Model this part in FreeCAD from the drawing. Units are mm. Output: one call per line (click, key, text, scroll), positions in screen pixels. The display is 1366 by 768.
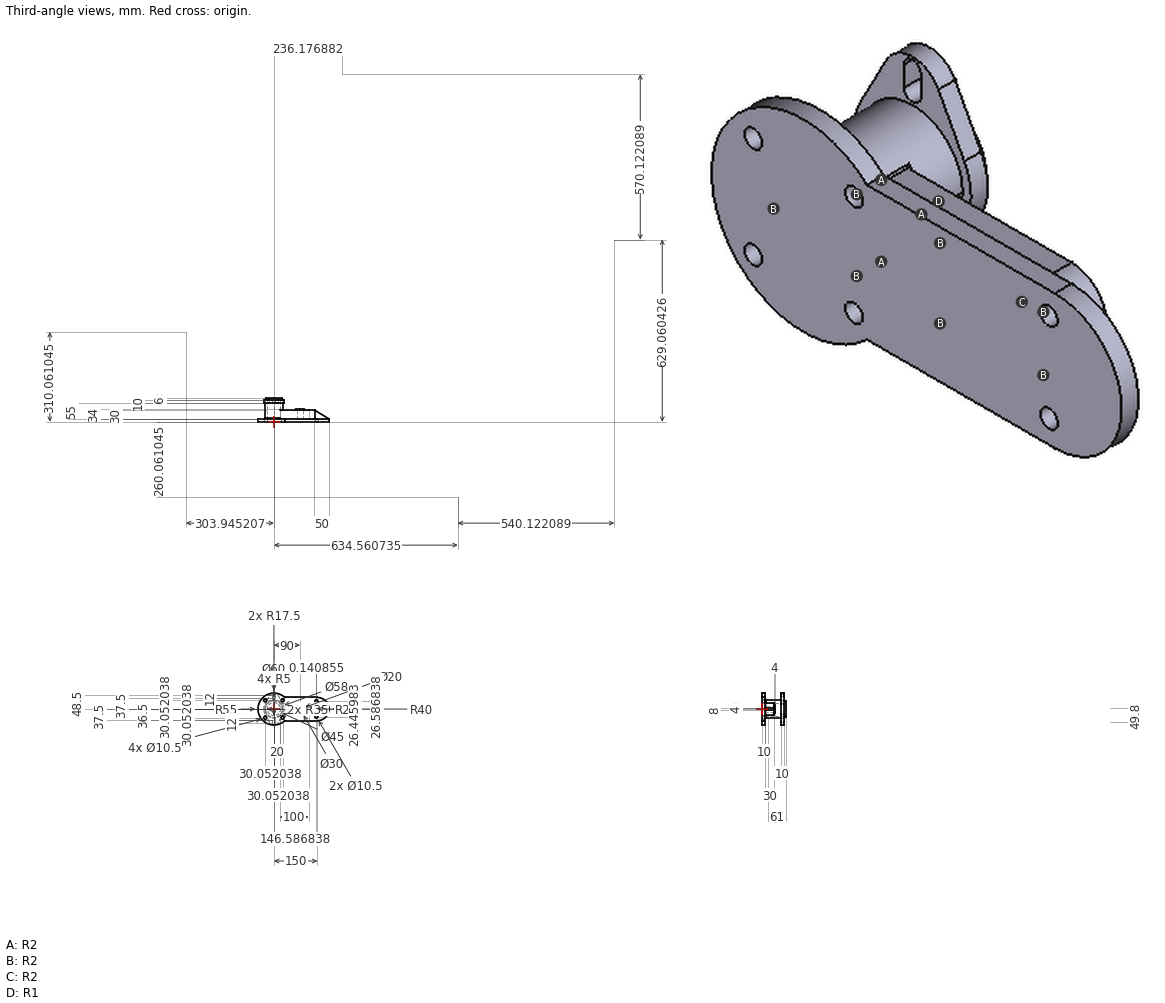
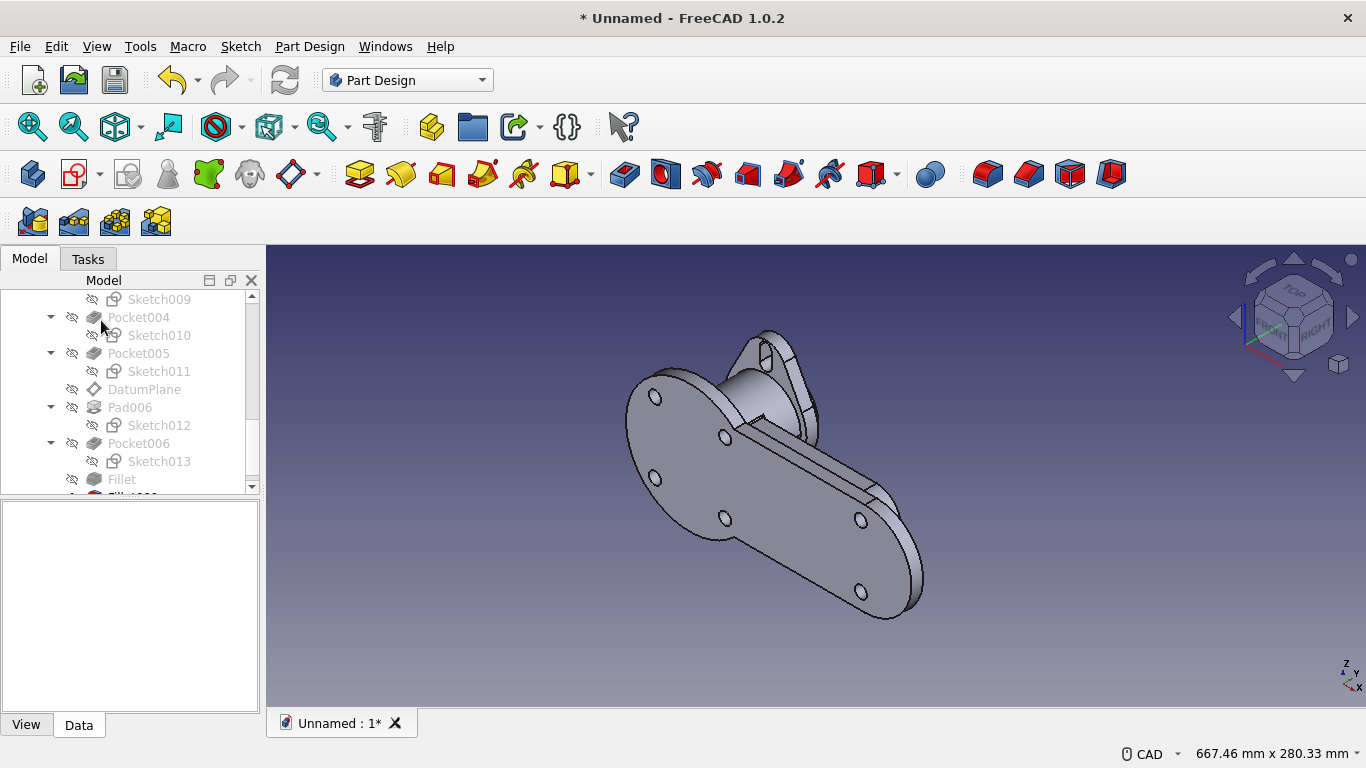
key(2)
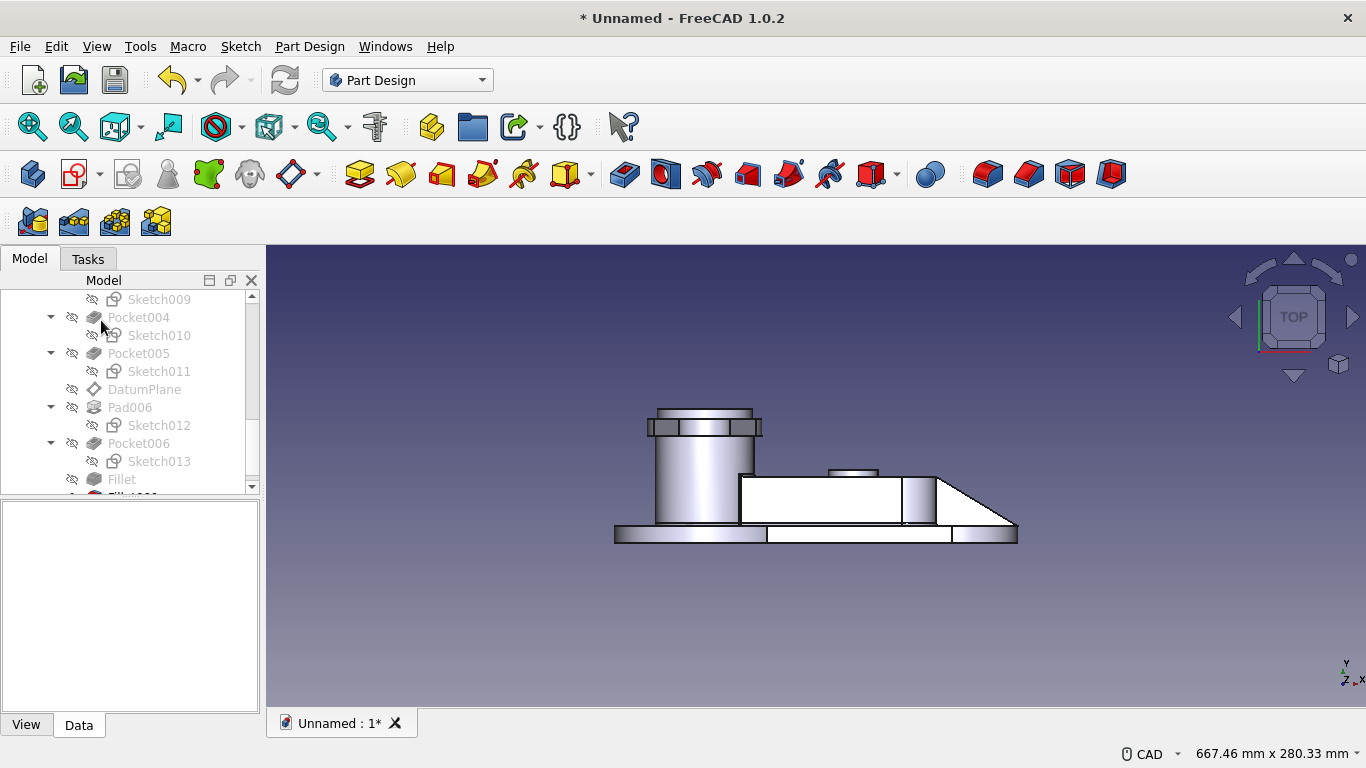
click(33, 128)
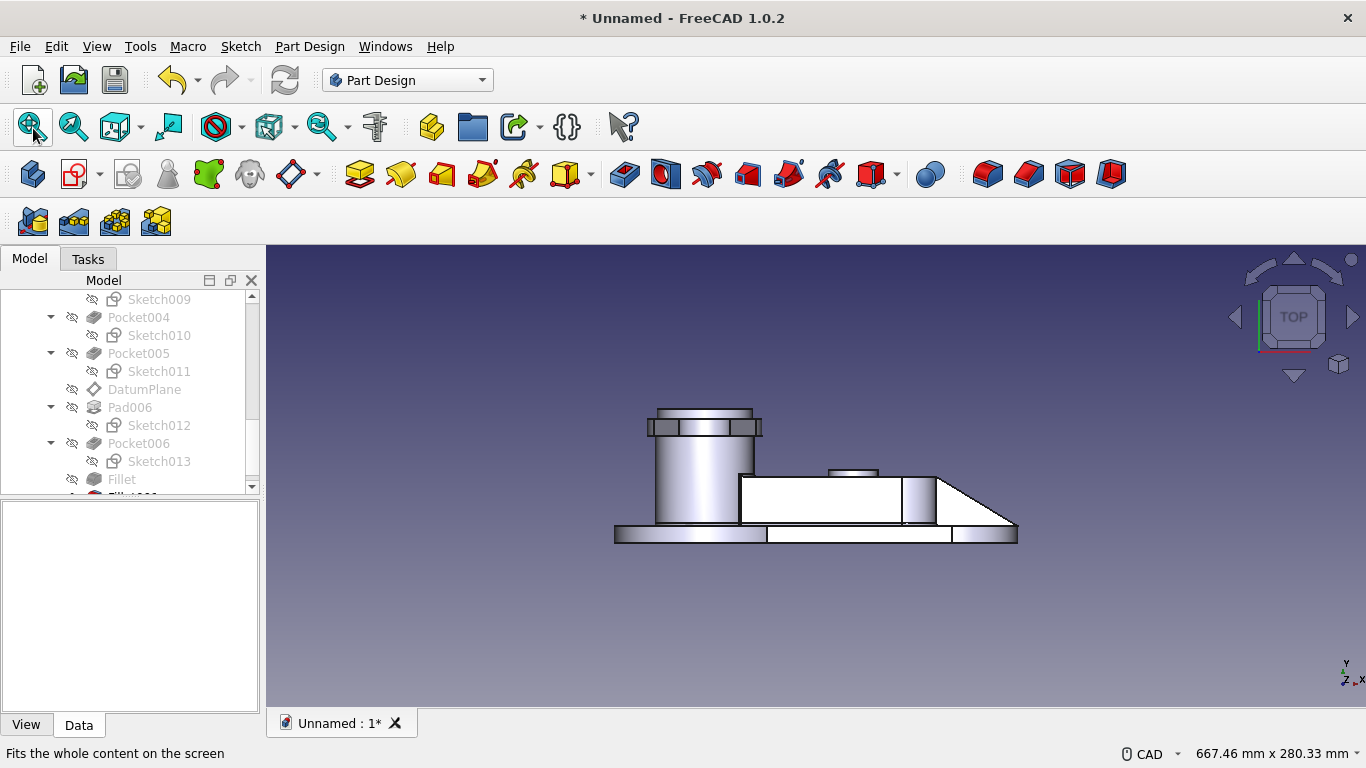
key(1)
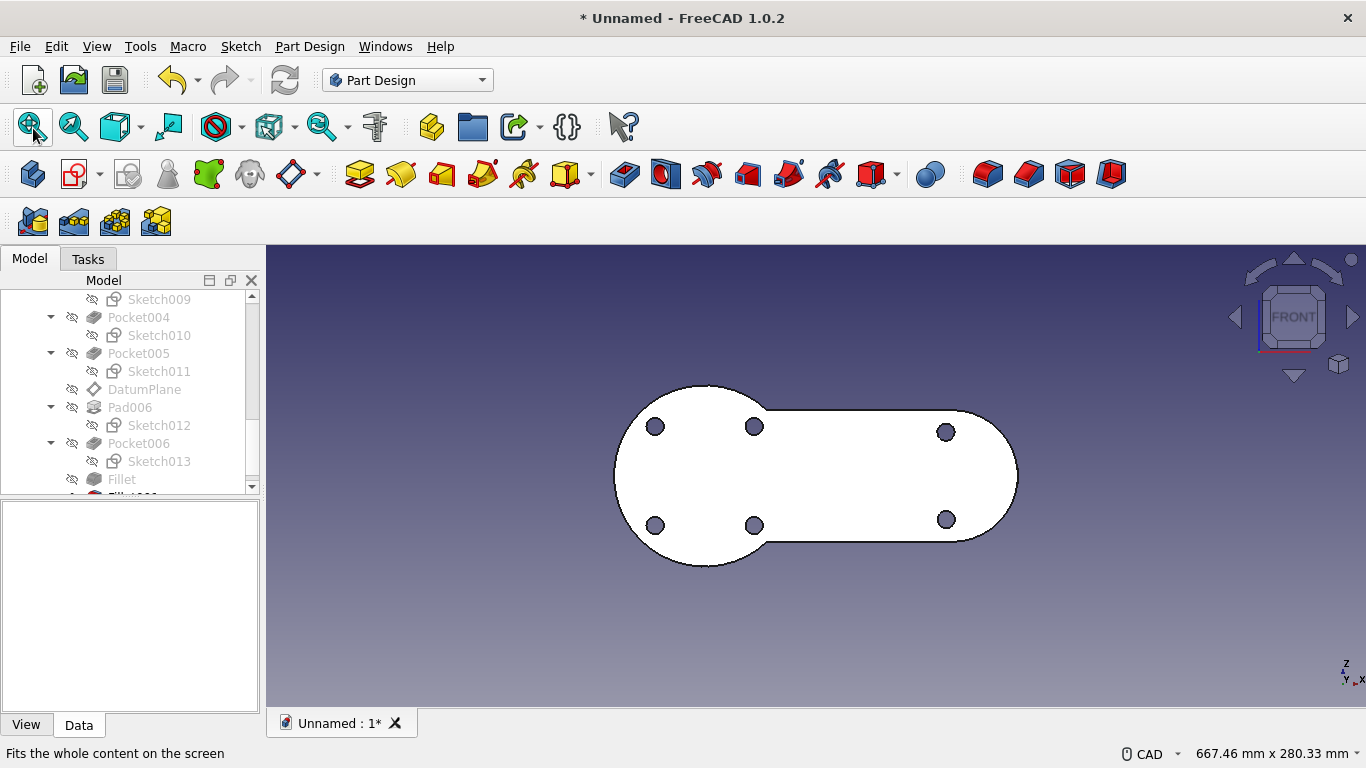
click(33, 128)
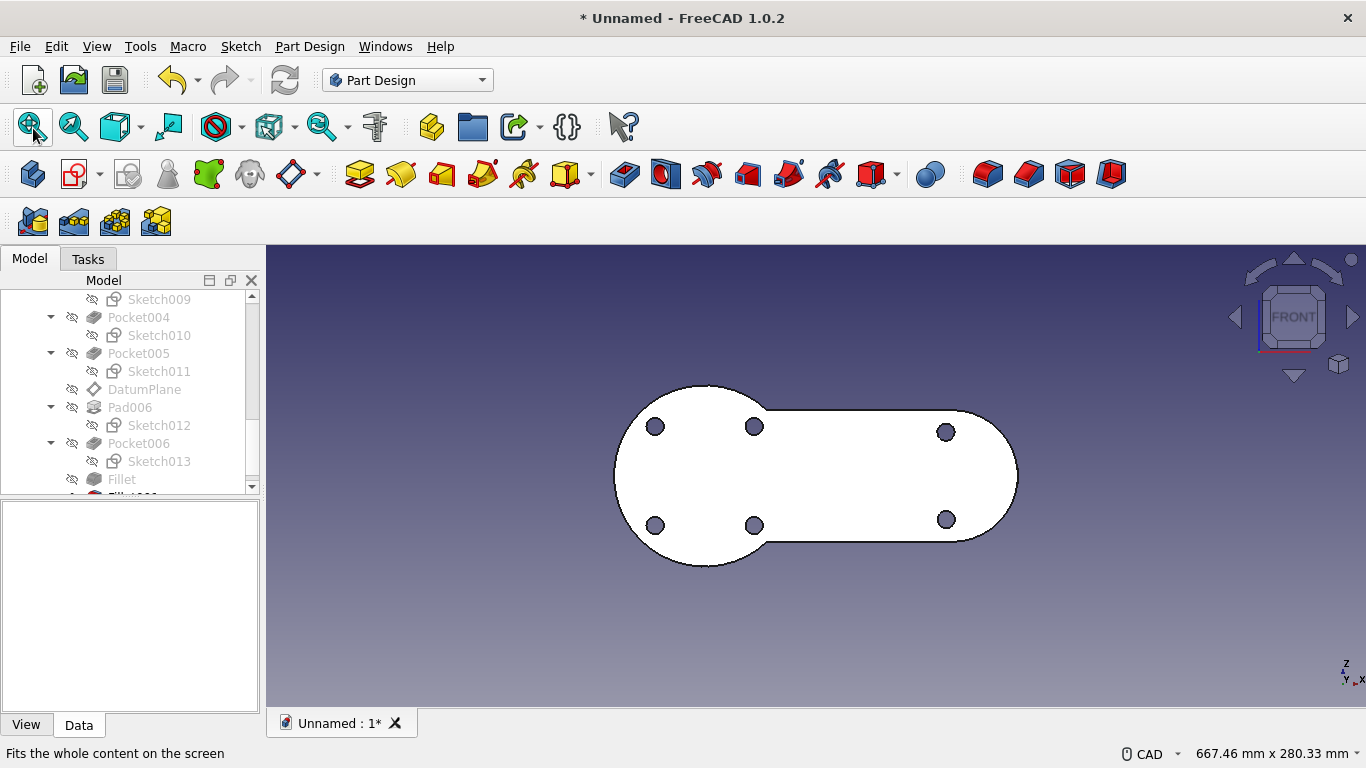
key(3)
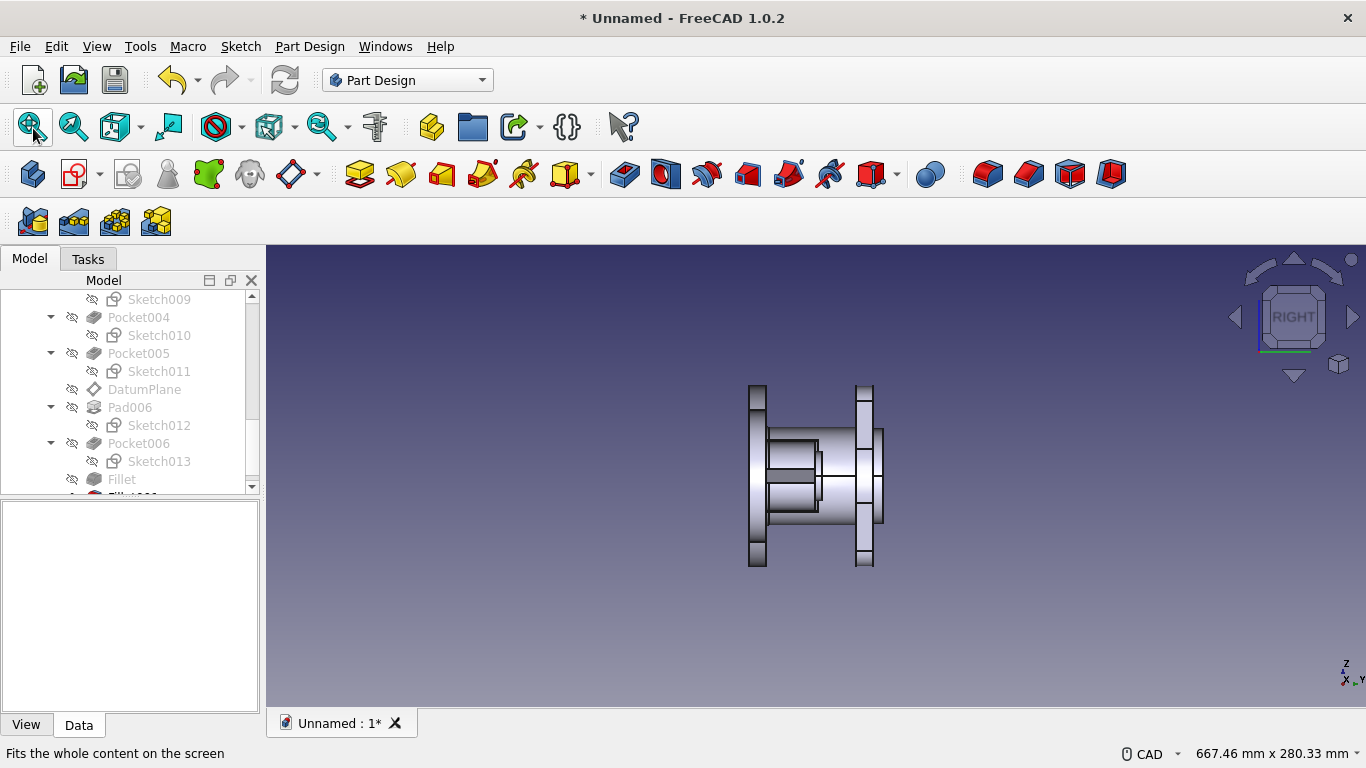
key(v)
key(f)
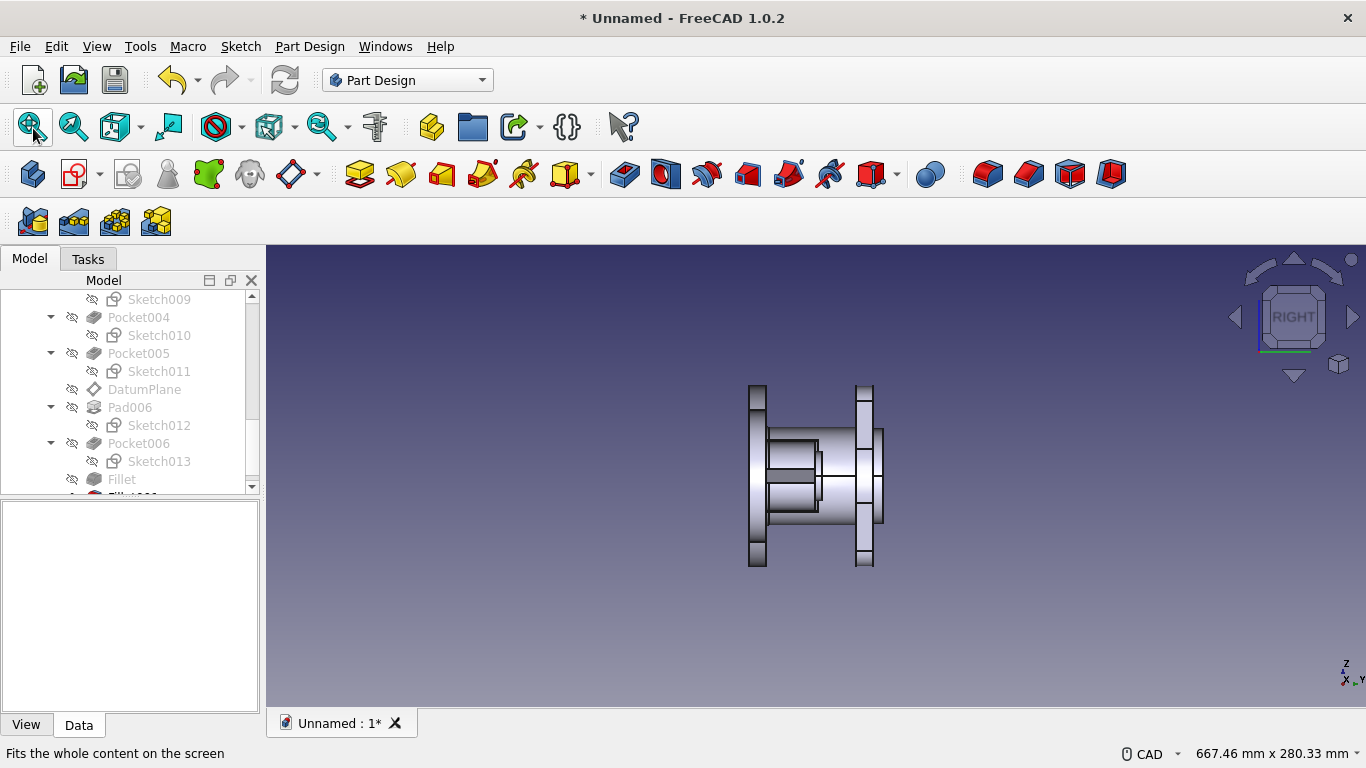
key(5)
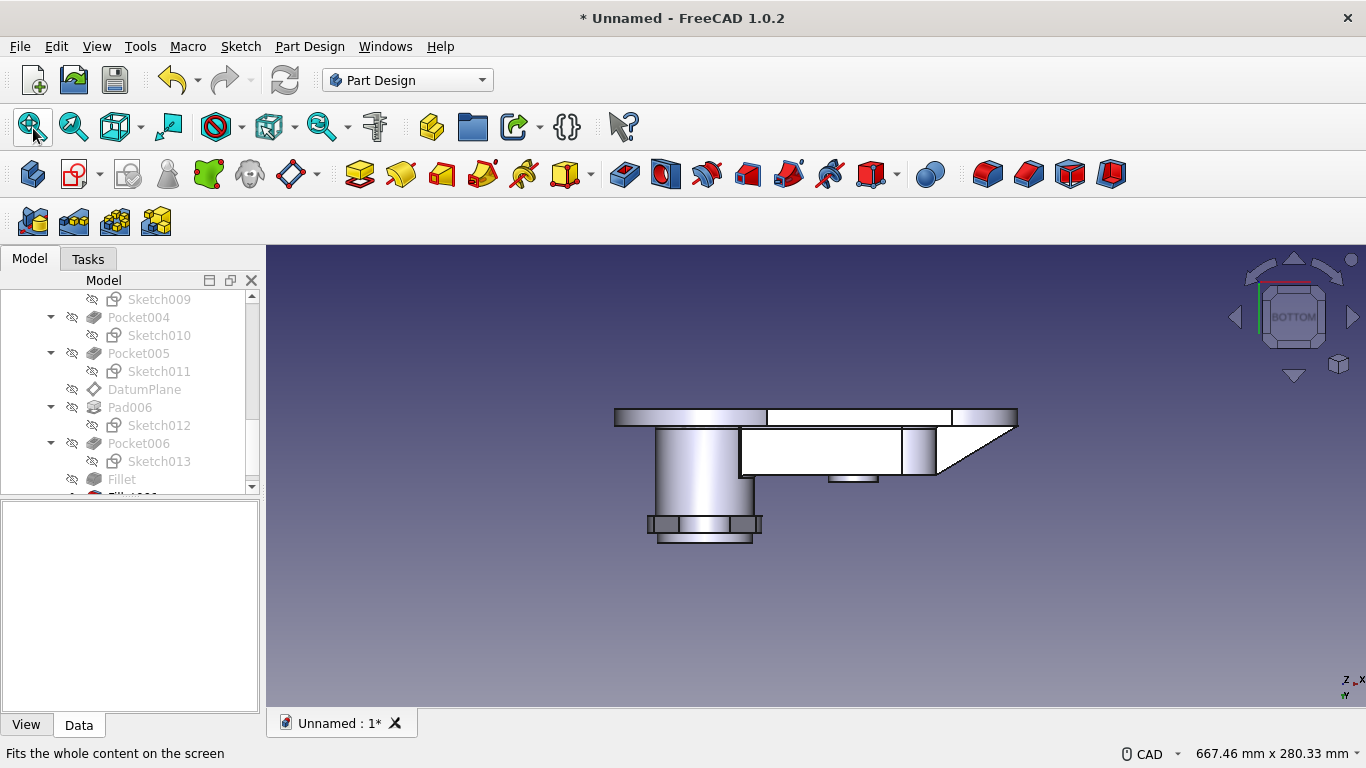
key(v)
key(f)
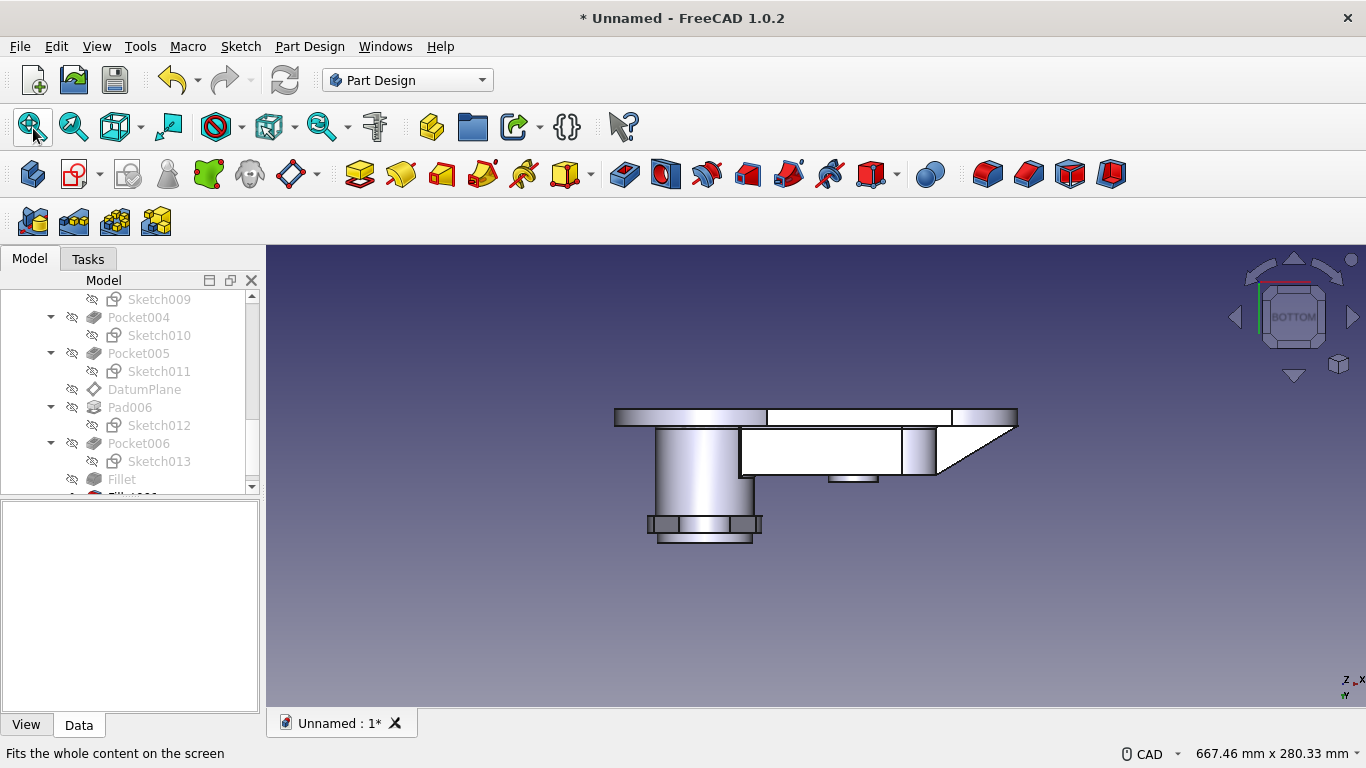
key(4)